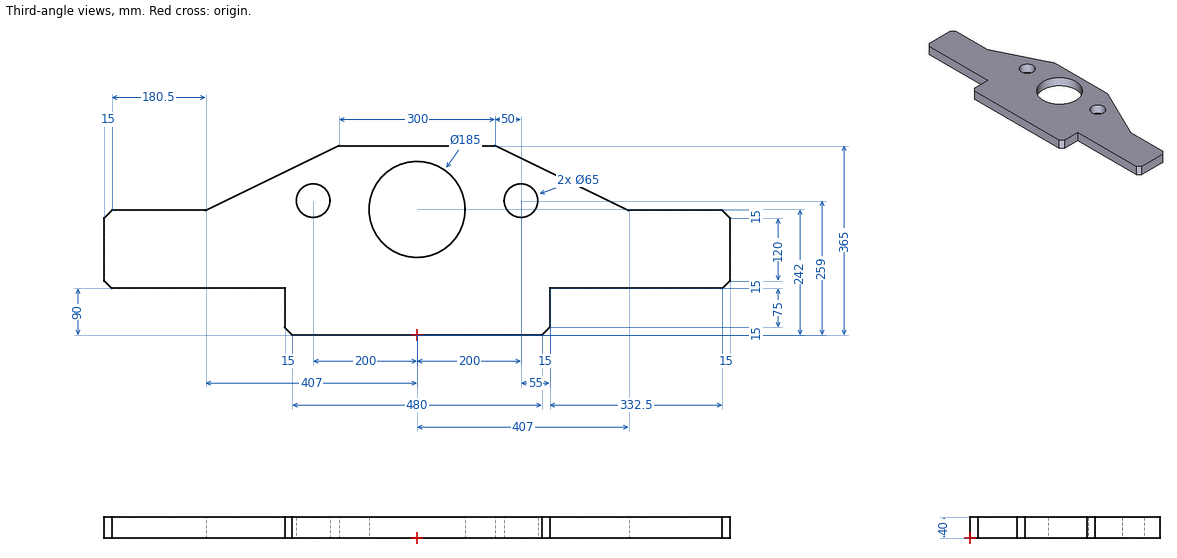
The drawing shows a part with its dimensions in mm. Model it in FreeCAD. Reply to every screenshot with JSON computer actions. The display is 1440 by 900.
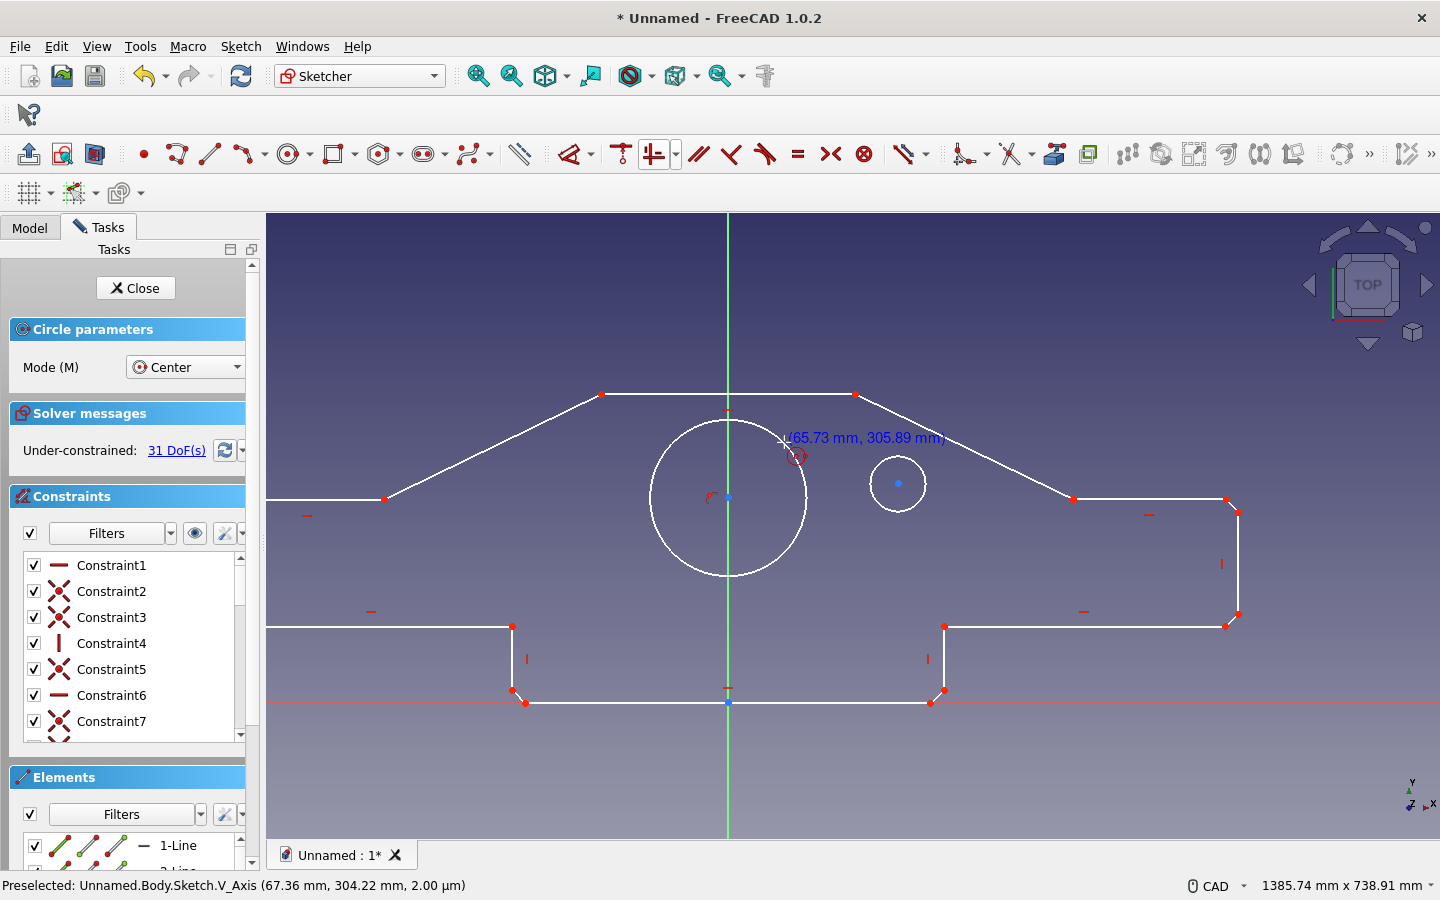
{"action": "left_click", "coordinate": [559, 483]}
{"action": "left_click", "coordinate": [578, 463]}
{"action": "key", "text": "Escape"}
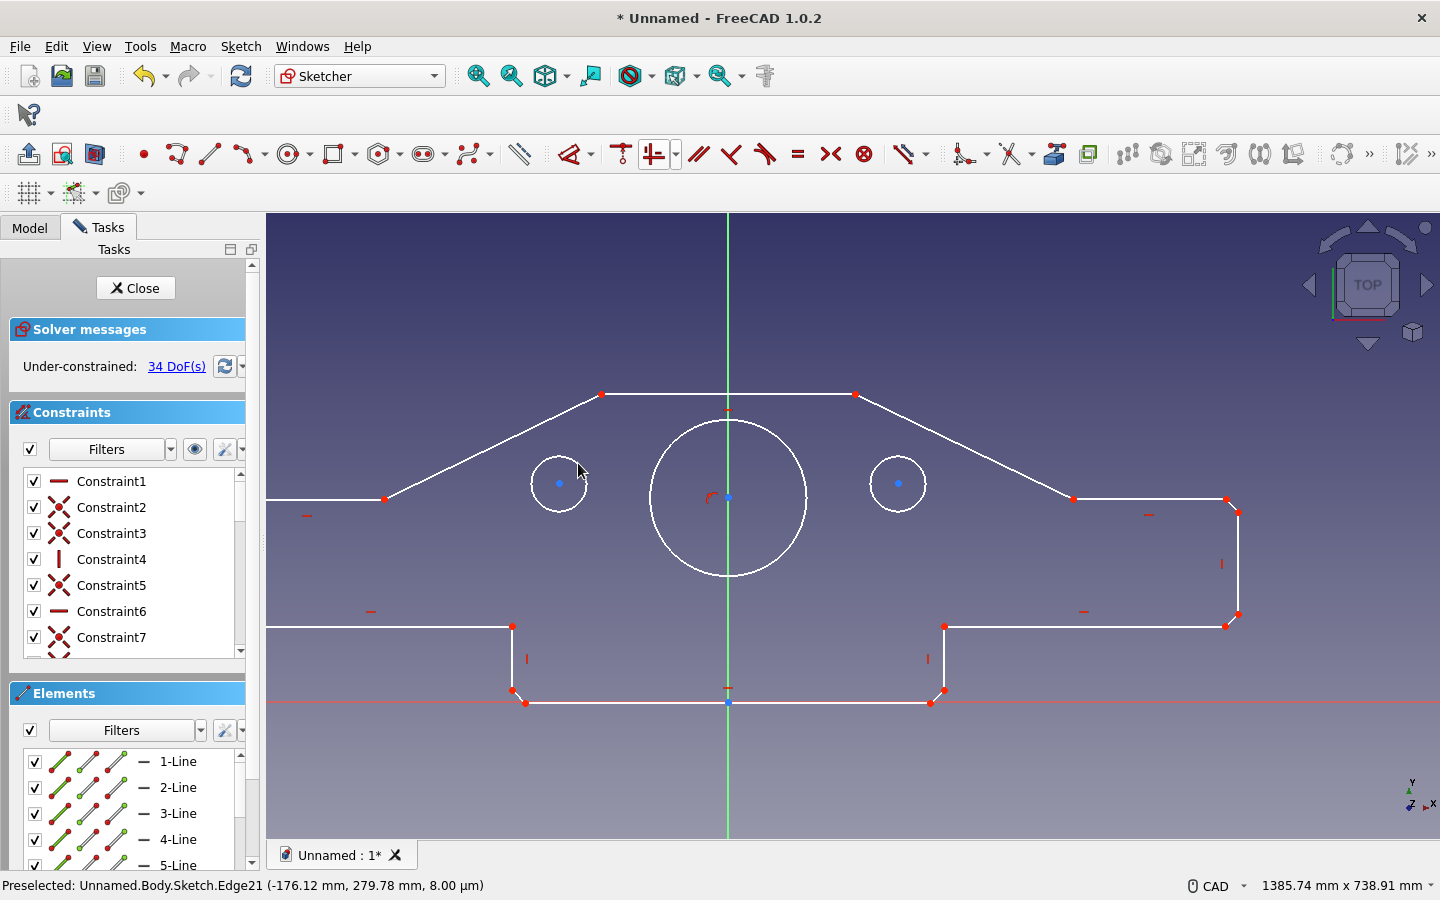
{"action": "left_click", "coordinate": [917, 464]}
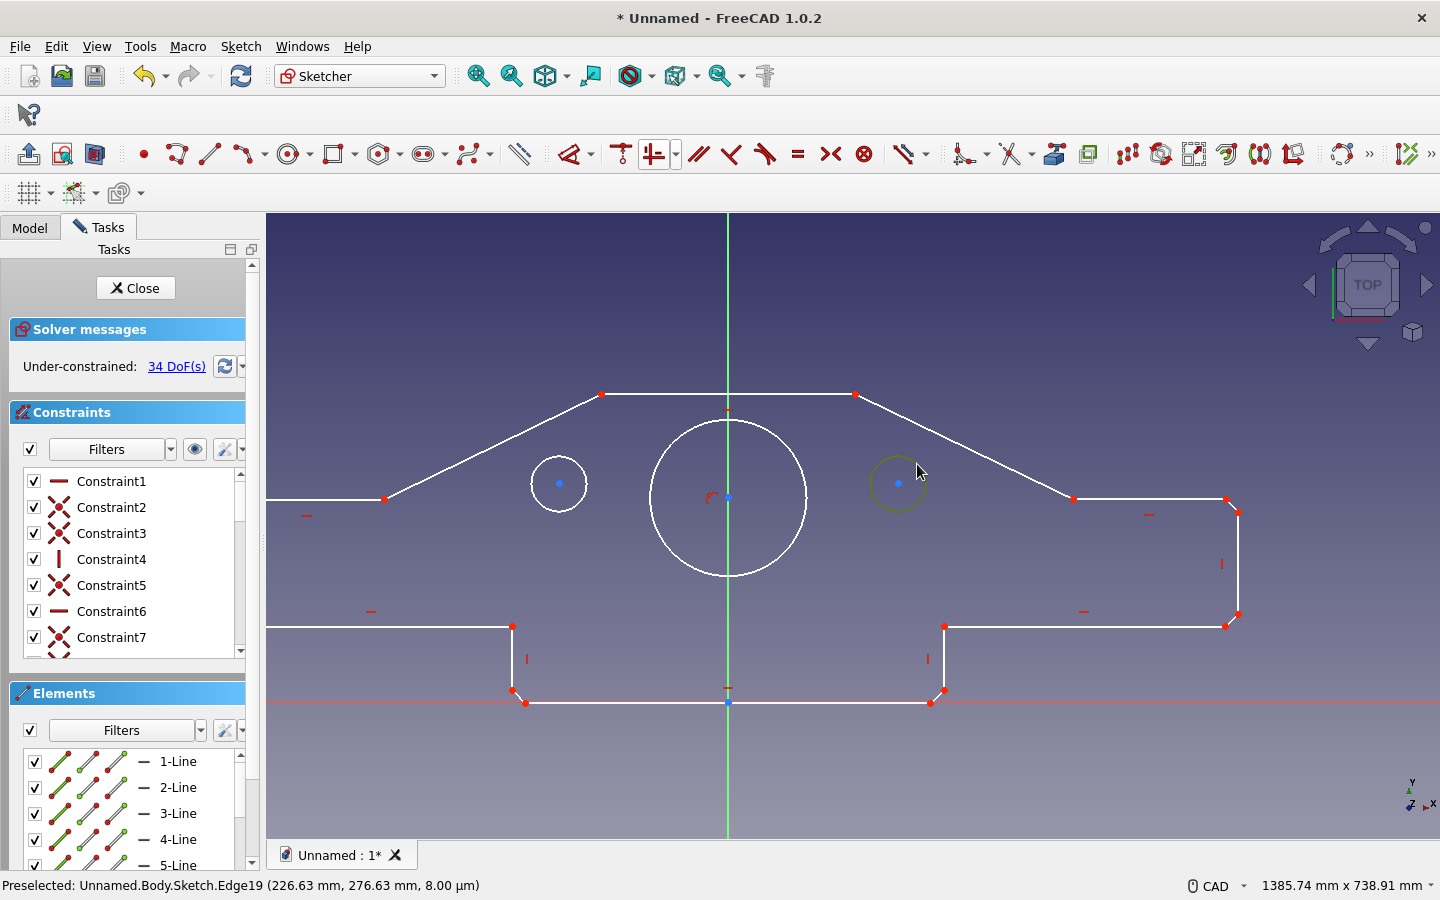
{"action": "left_click", "coordinate": [578, 464]}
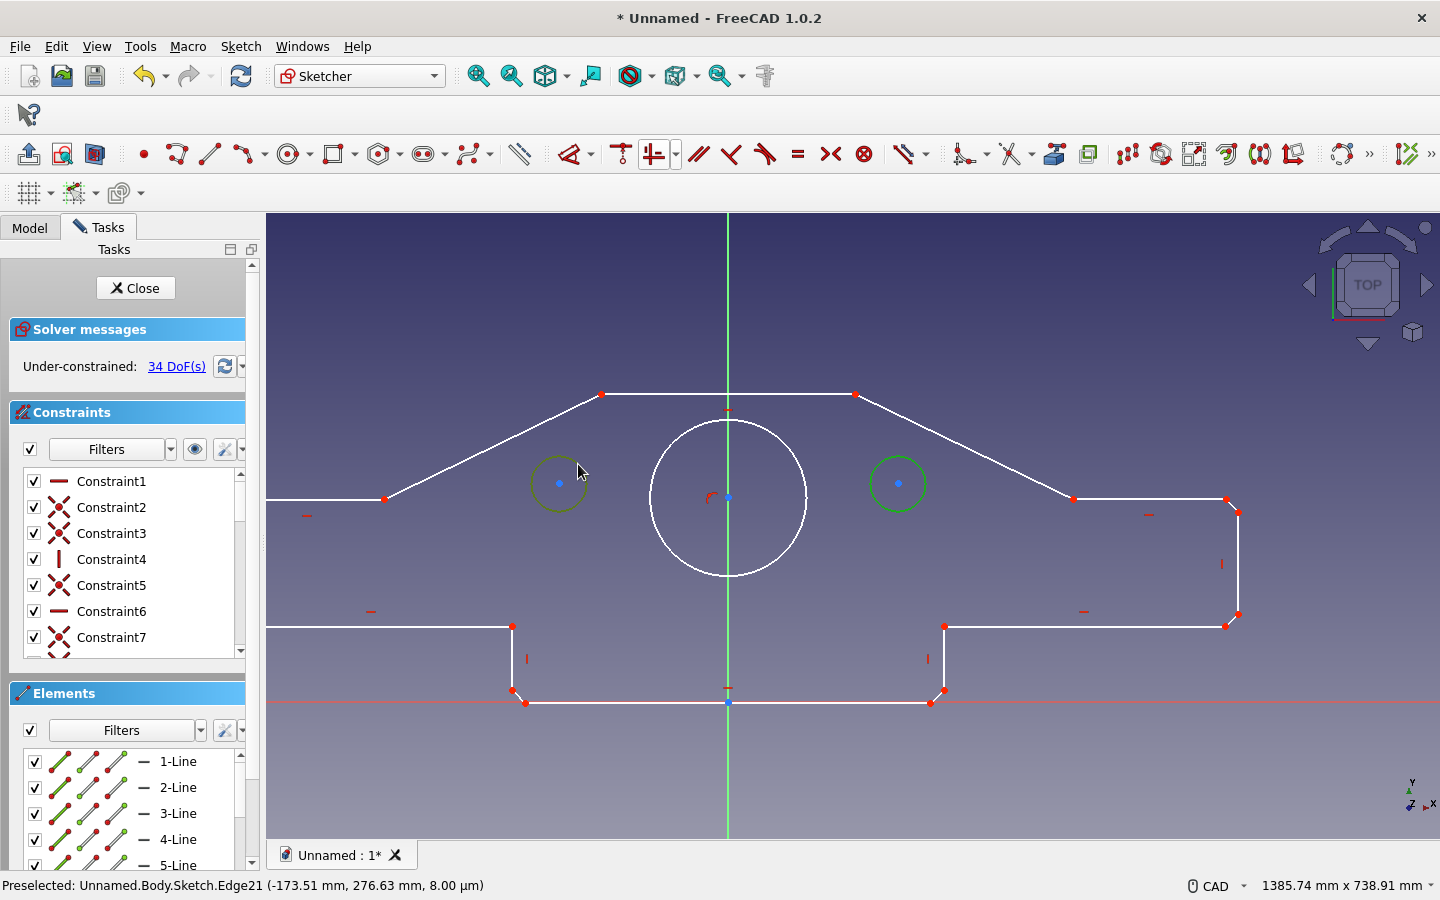
{"action": "left_click", "coordinate": [798, 154]}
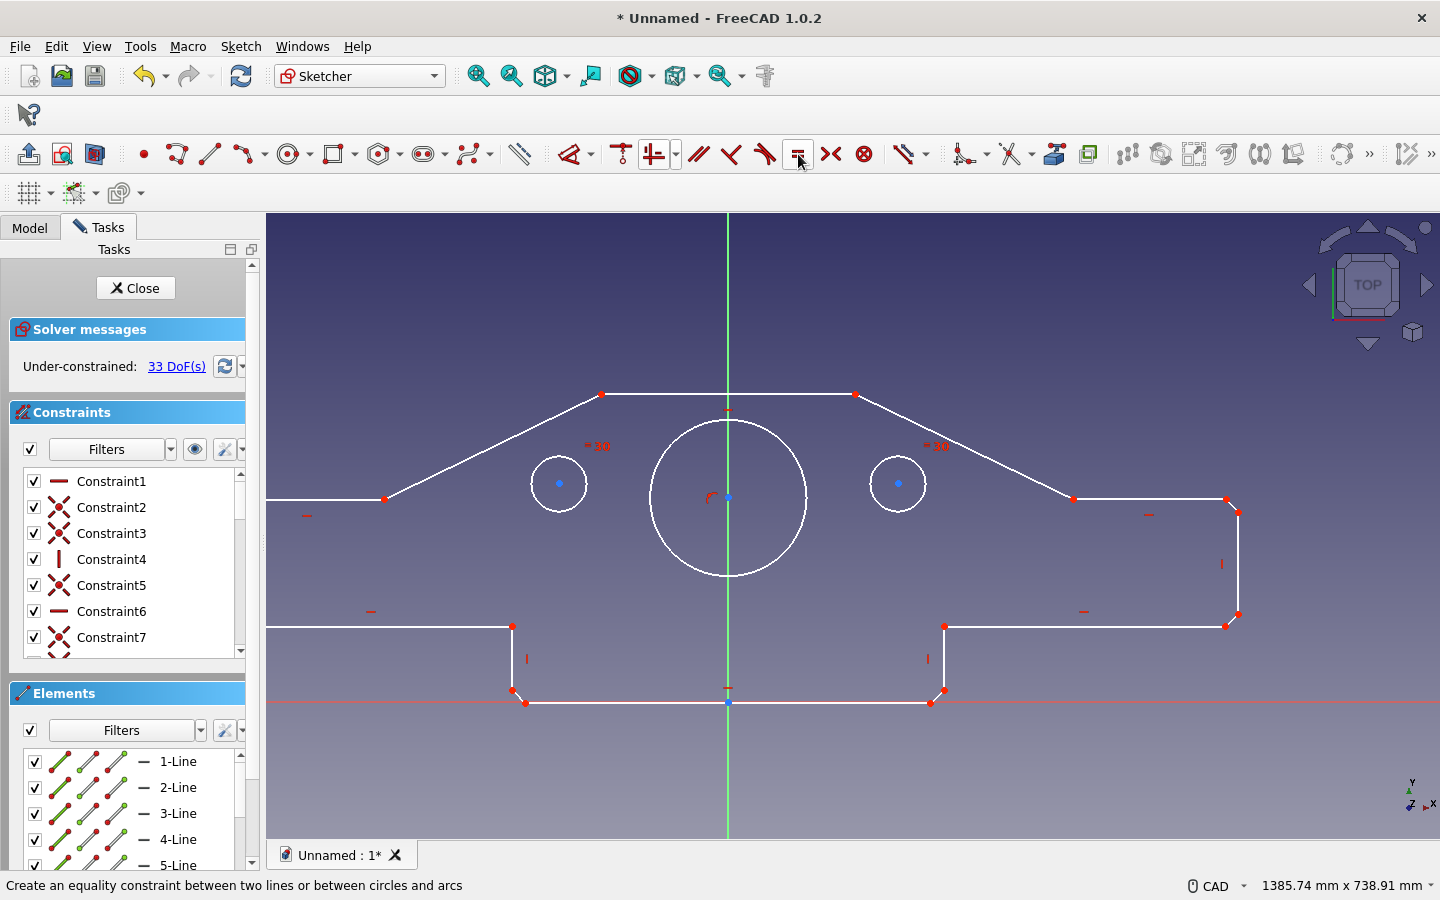
{"action": "left_click", "coordinate": [568, 154]}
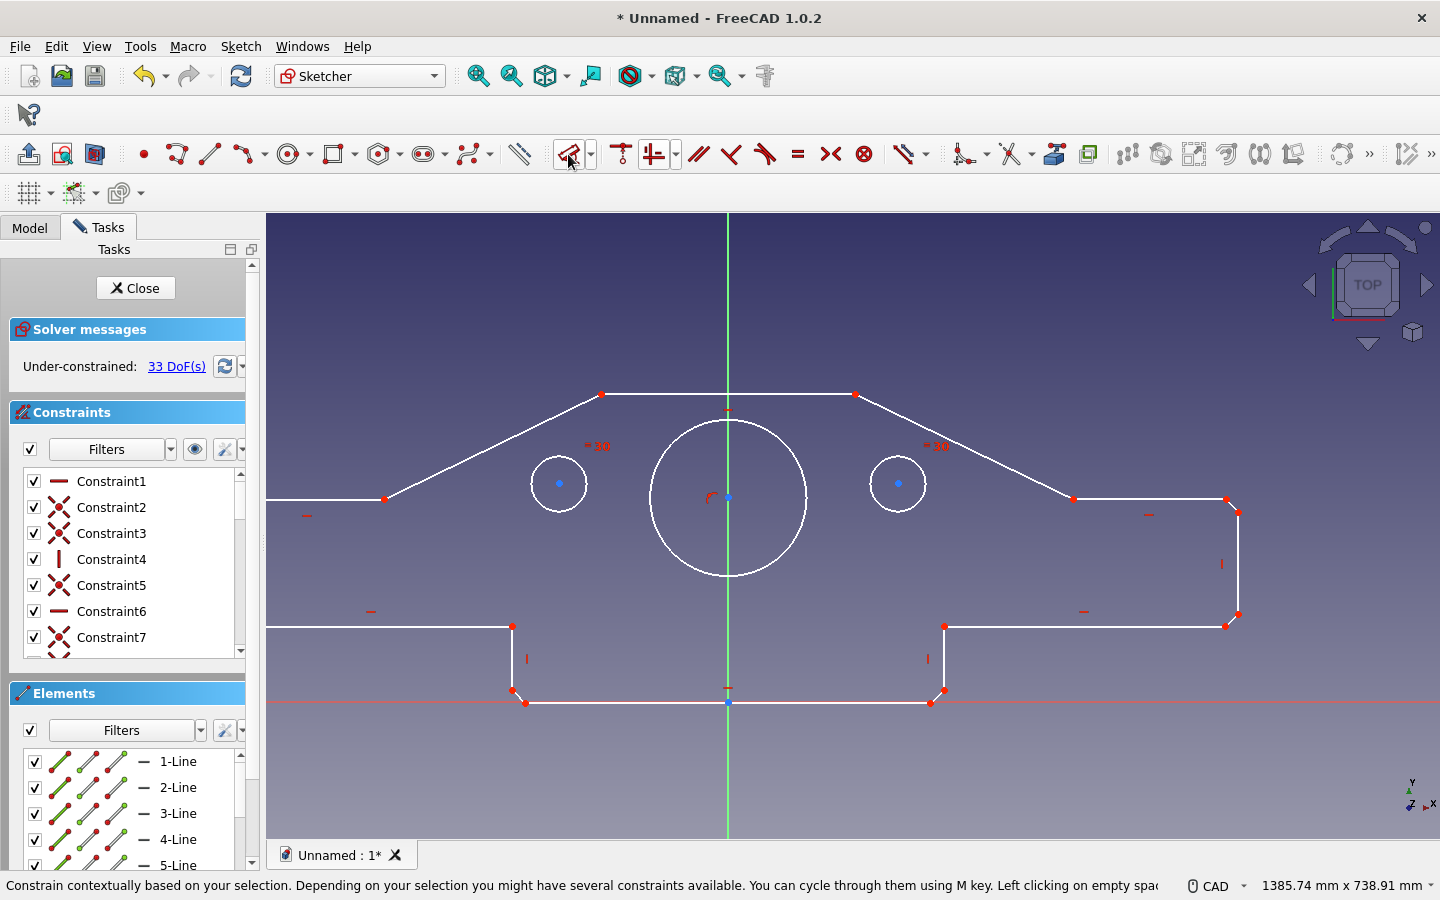
{"action": "left_click", "coordinate": [917, 464]}
{"action": "left_click", "coordinate": [955, 466]}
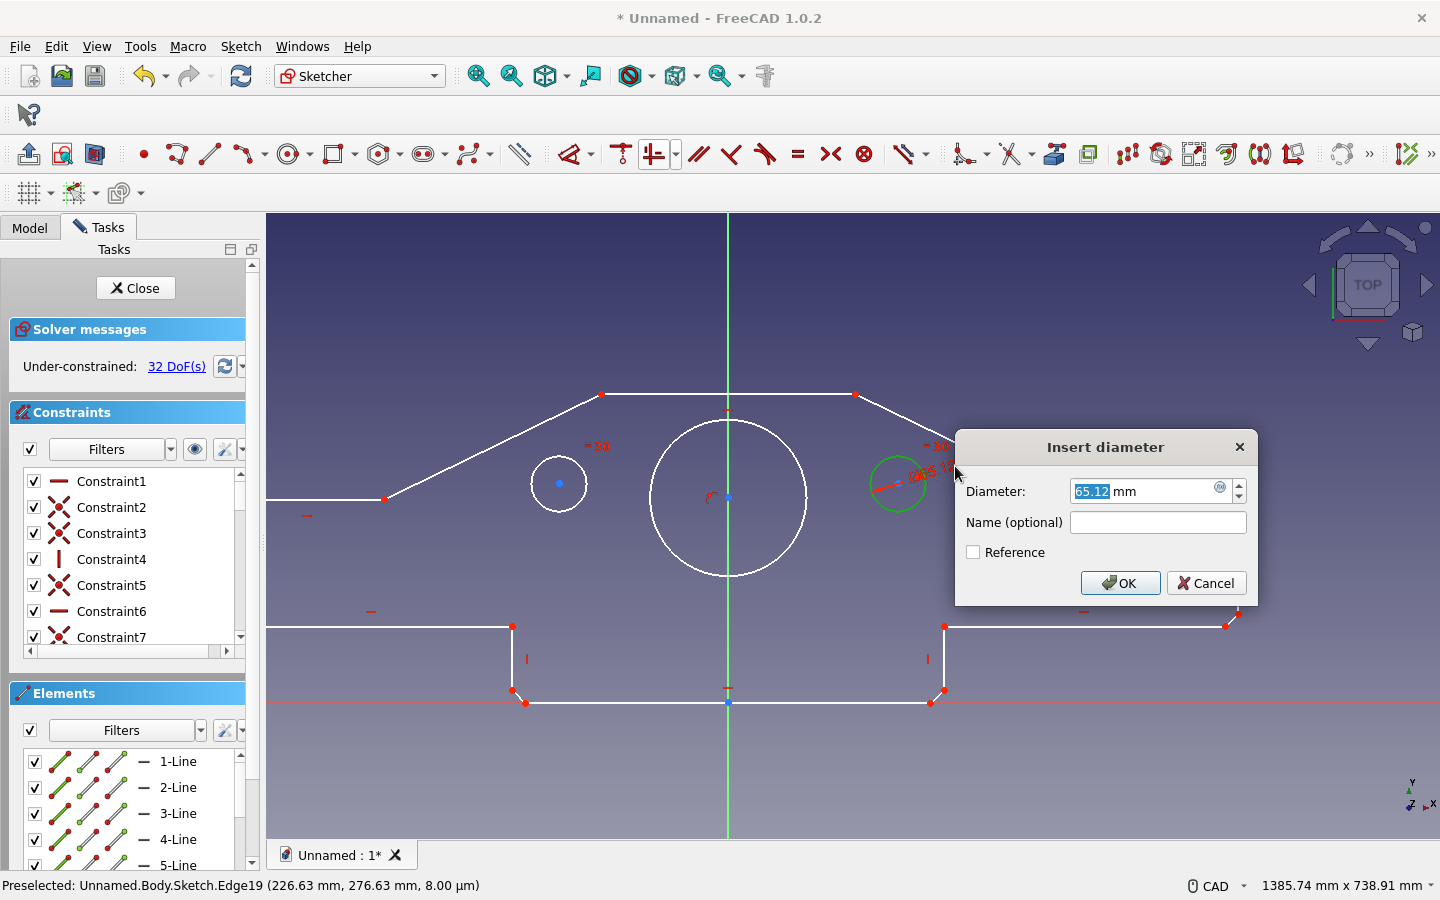
{"action": "type", "text": "65"}
{"action": "key", "text": "Return"}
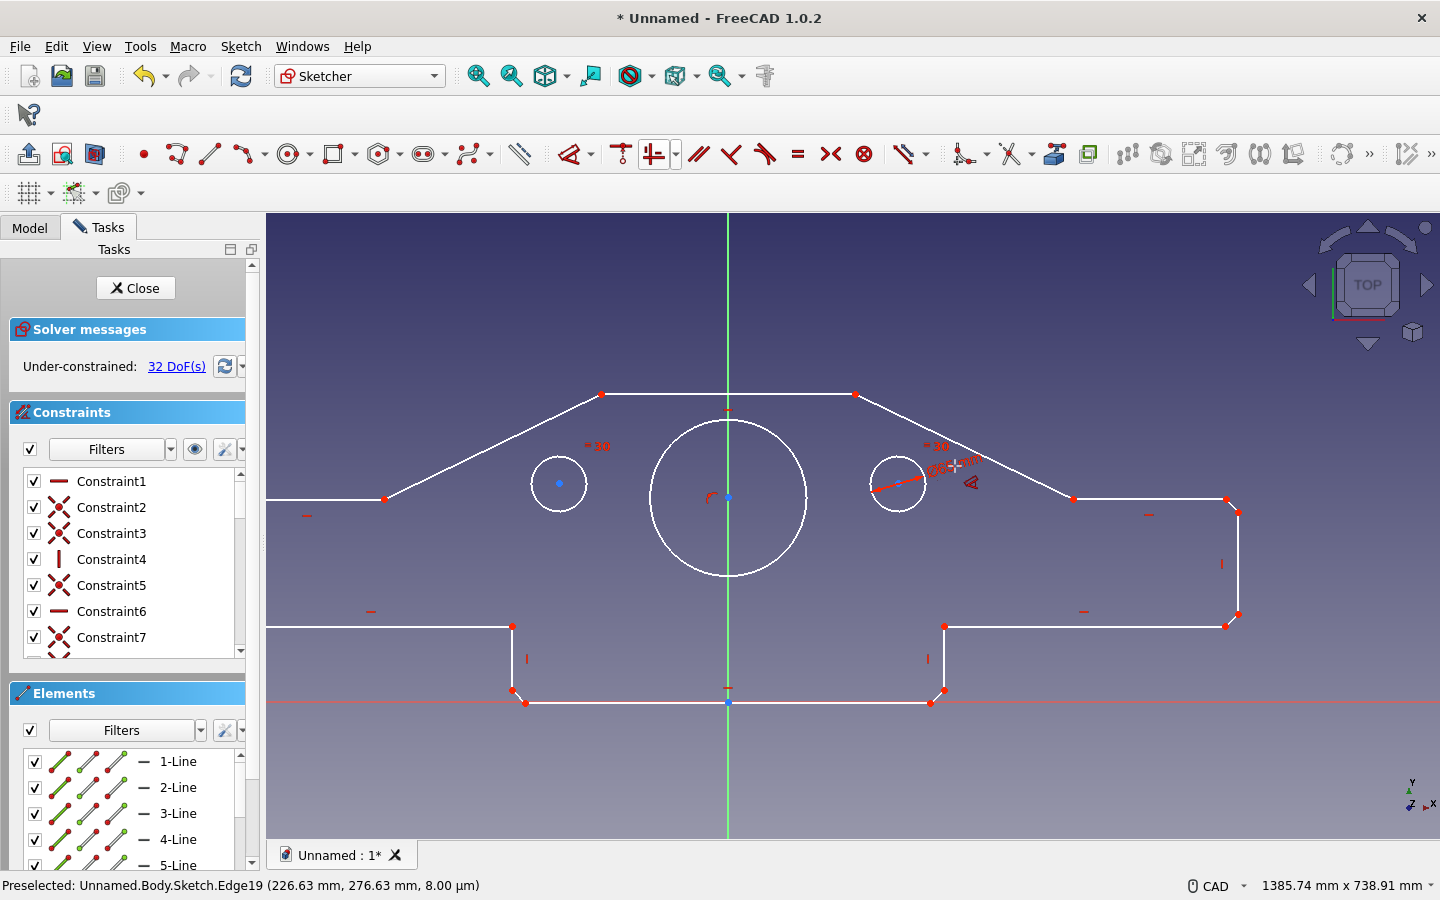
{"action": "left_click", "coordinate": [783, 442]}
{"action": "left_click", "coordinate": [805, 419]}